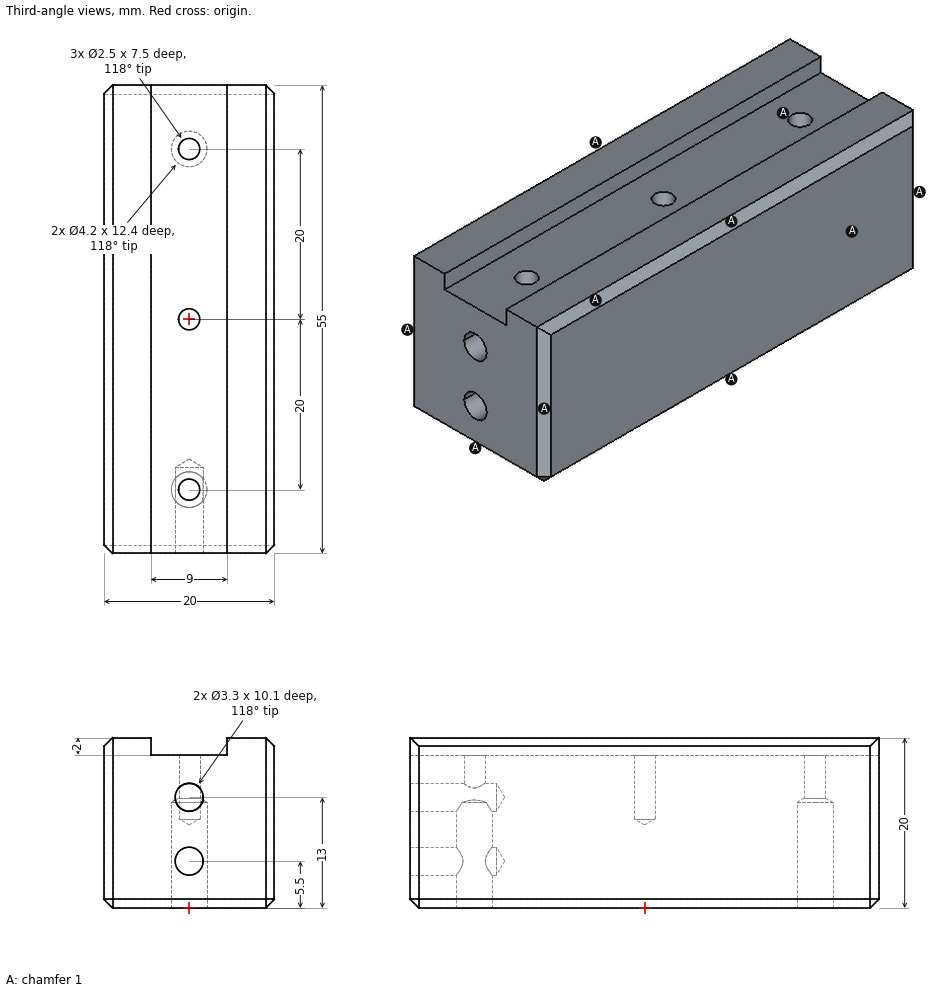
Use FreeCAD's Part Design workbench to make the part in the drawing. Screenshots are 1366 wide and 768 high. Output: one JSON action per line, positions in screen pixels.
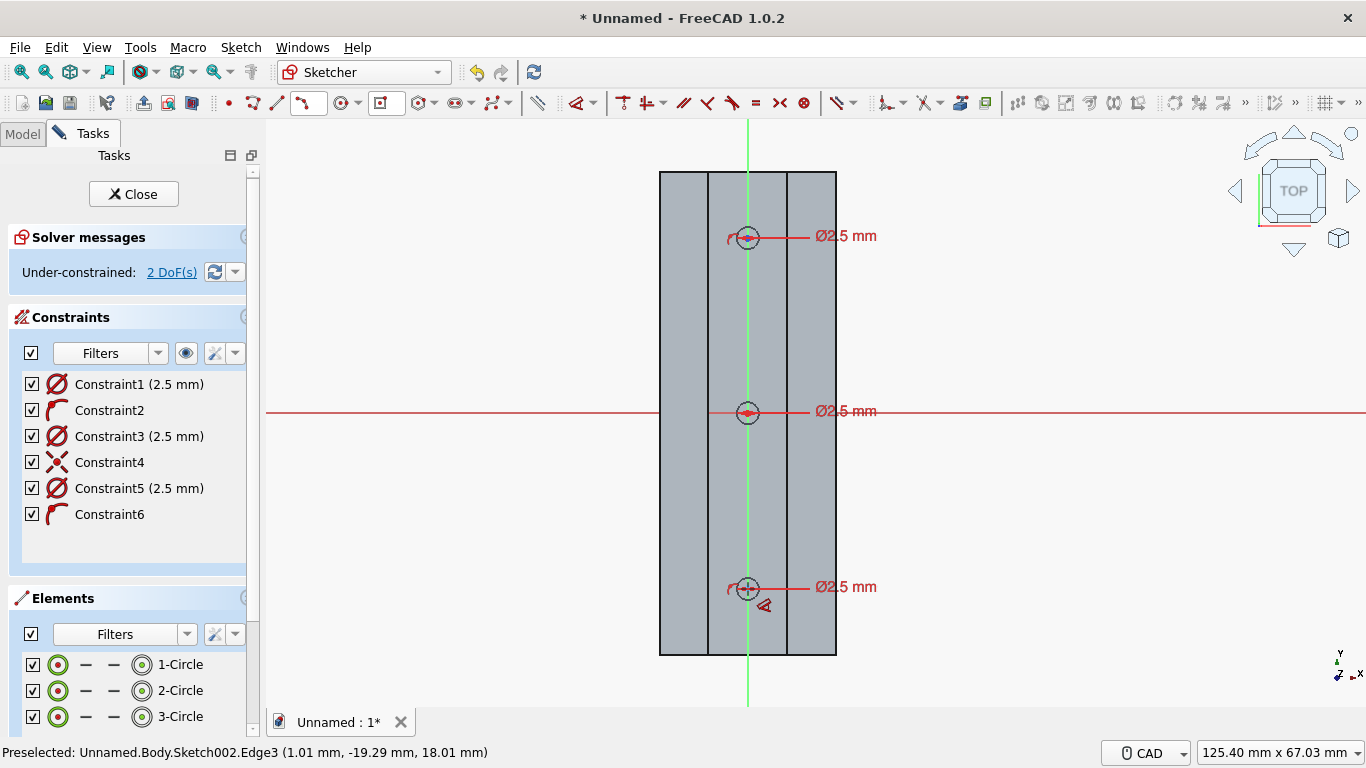
{"action": "left_click", "coordinate": [748, 238]}
{"action": "left_click", "coordinate": [782, 326]}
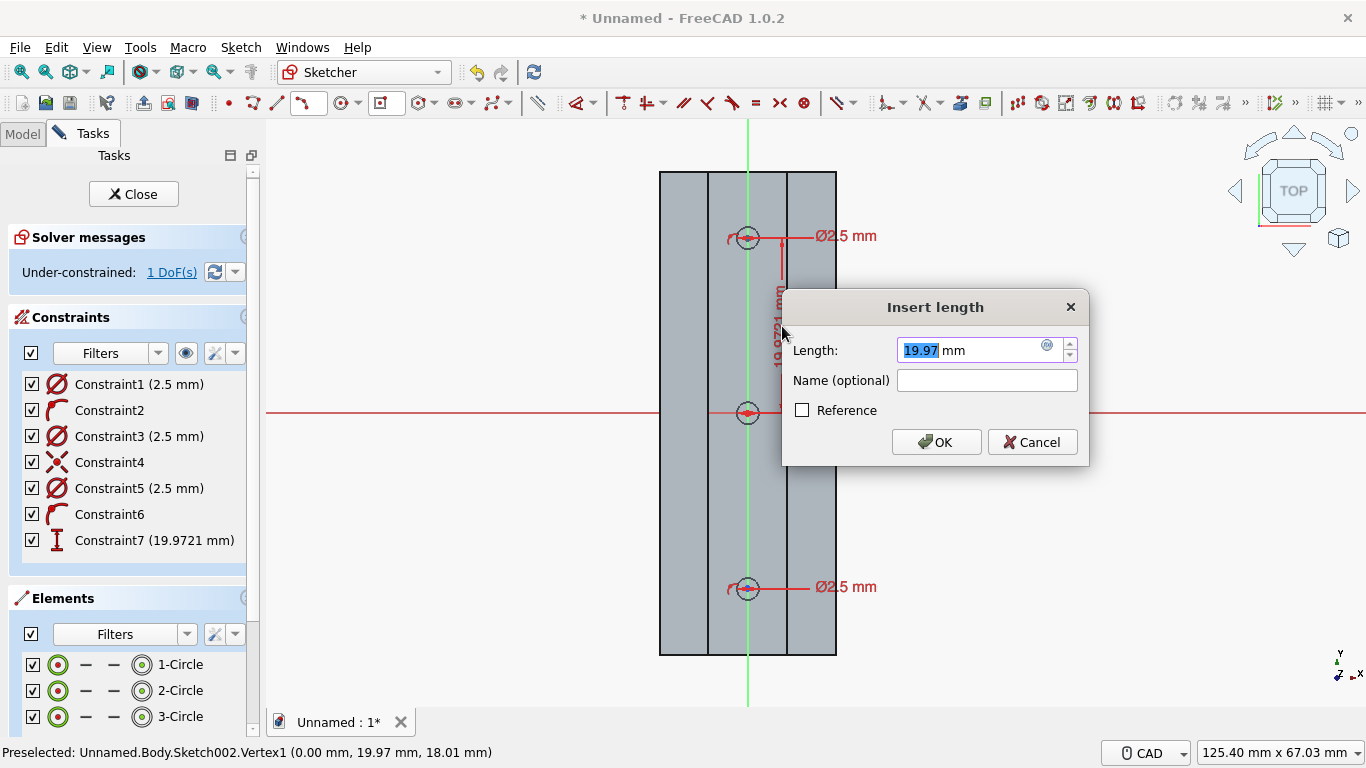
{"action": "type", "text": "20"}
{"action": "key", "text": "Return"}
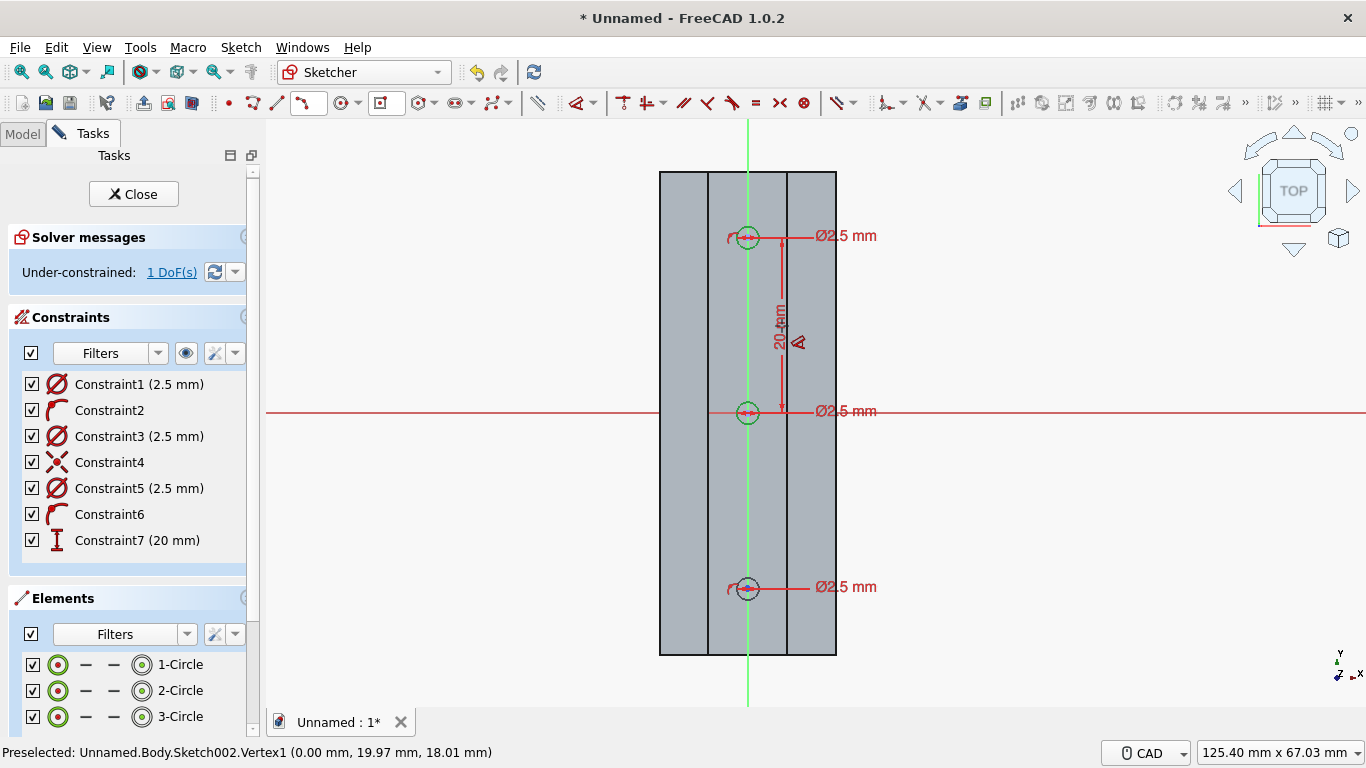
{"action": "left_click", "coordinate": [748, 589]}
{"action": "left_click", "coordinate": [782, 501]}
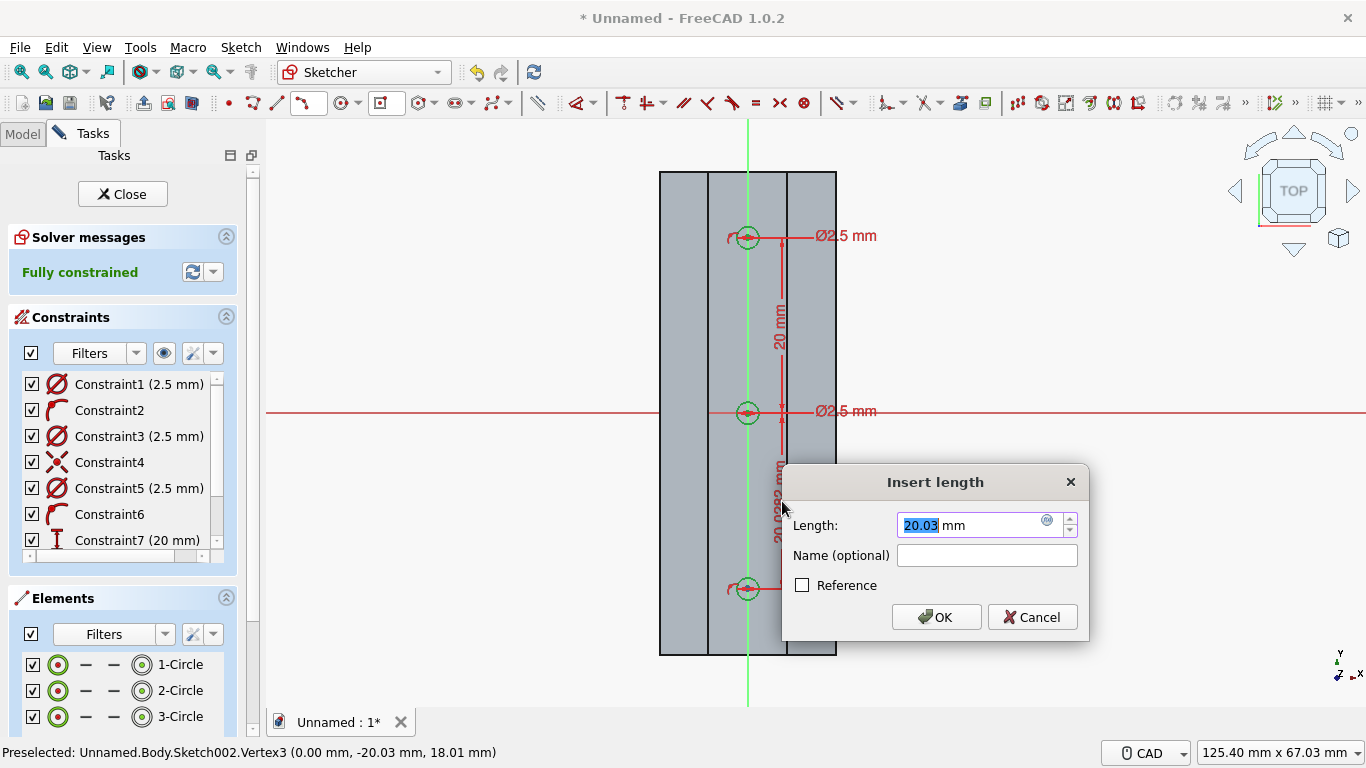
{"action": "type", "text": "20"}
{"action": "key", "text": "Return"}
{"action": "key", "text": "Escape"}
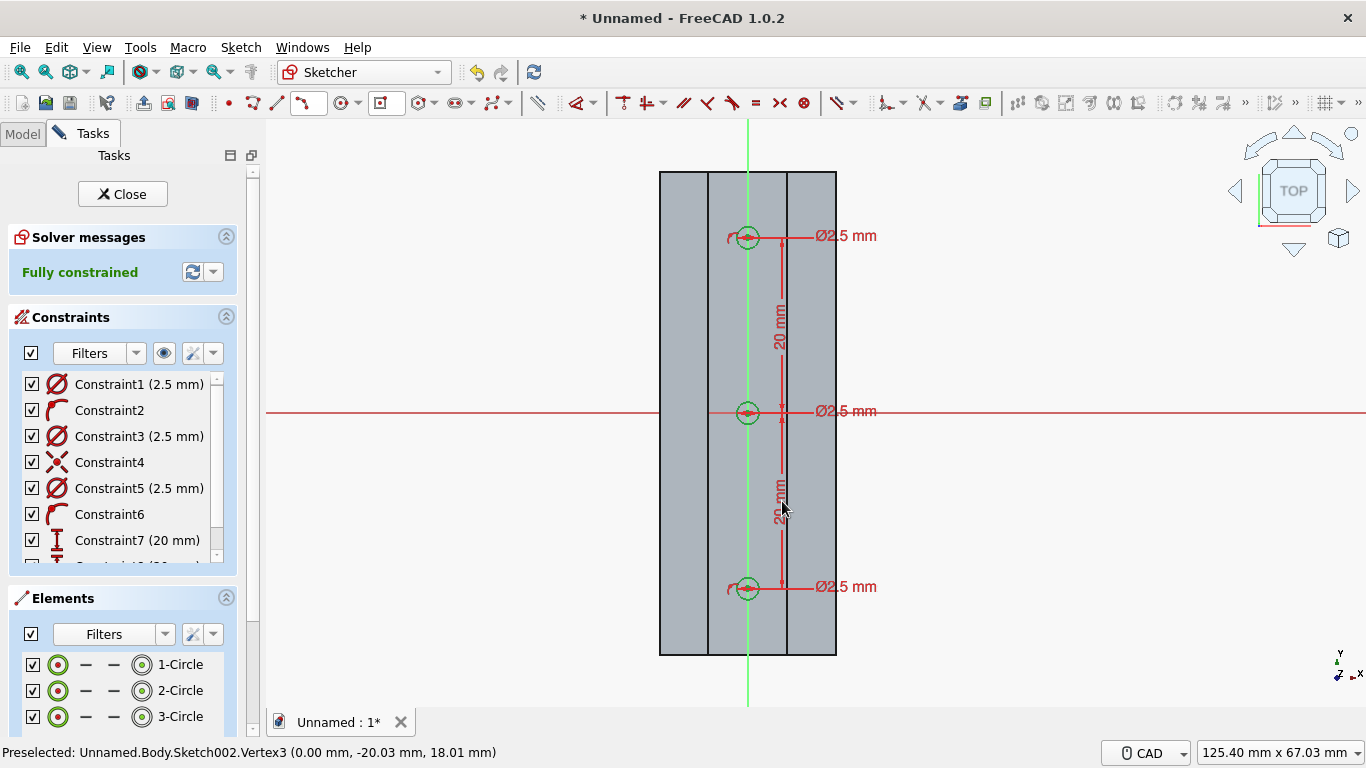
{"action": "left_click", "coordinate": [123, 194]}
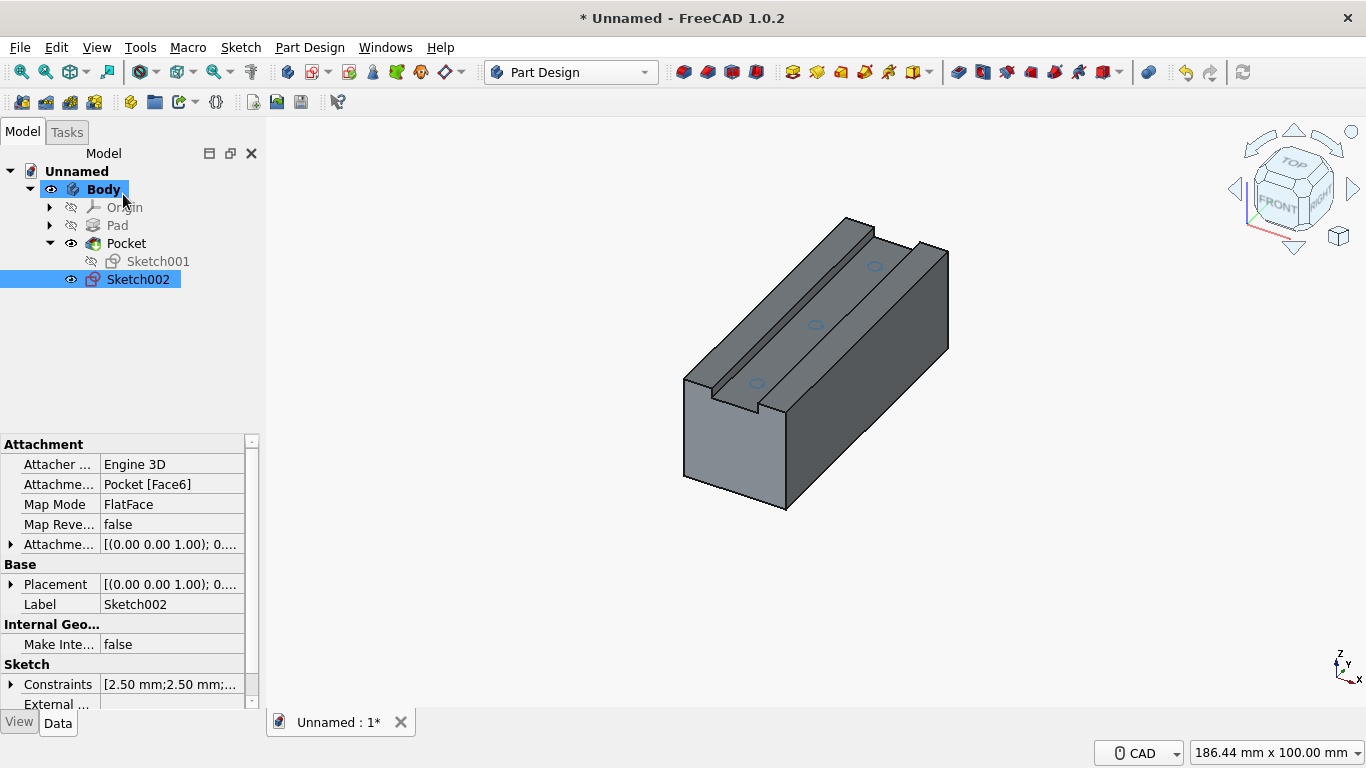
{"action": "left_click", "coordinate": [984, 72]}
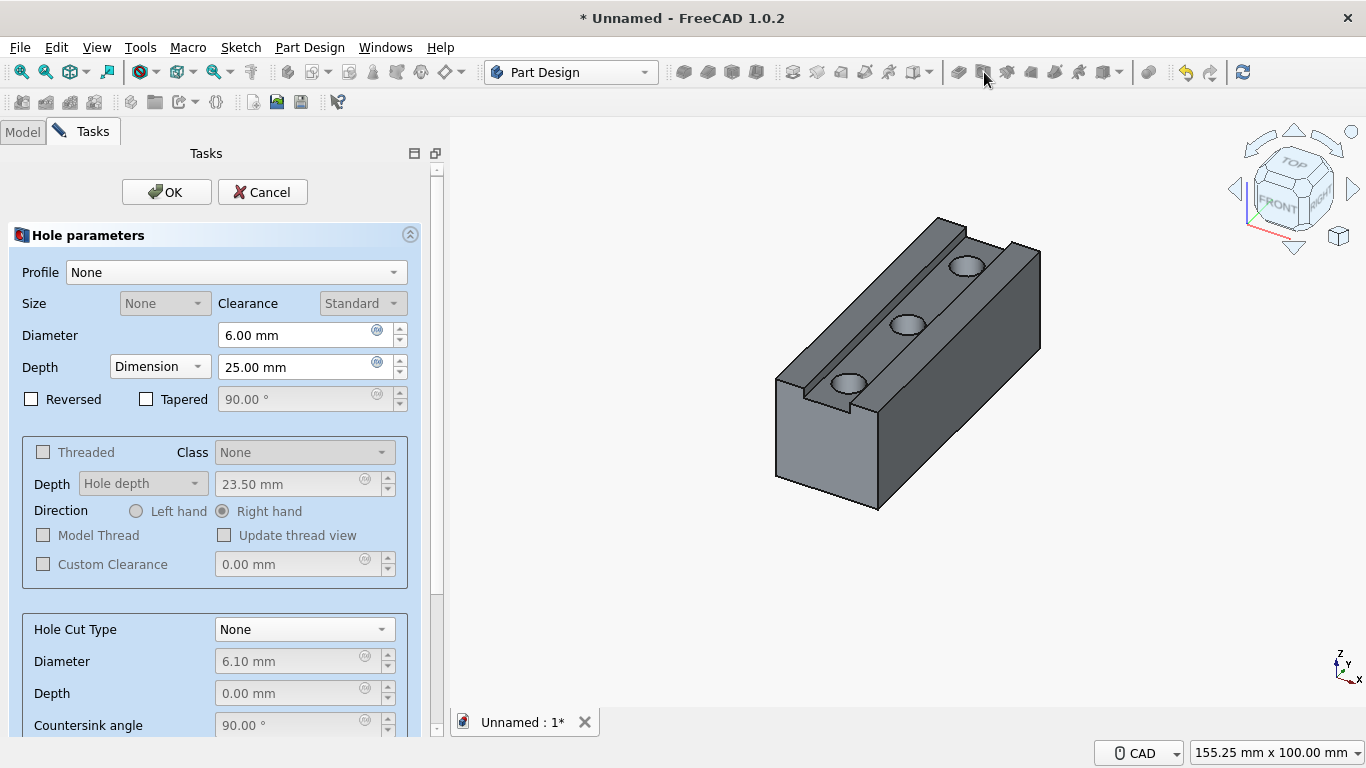
{"action": "triple_click", "coordinate": [305, 335]}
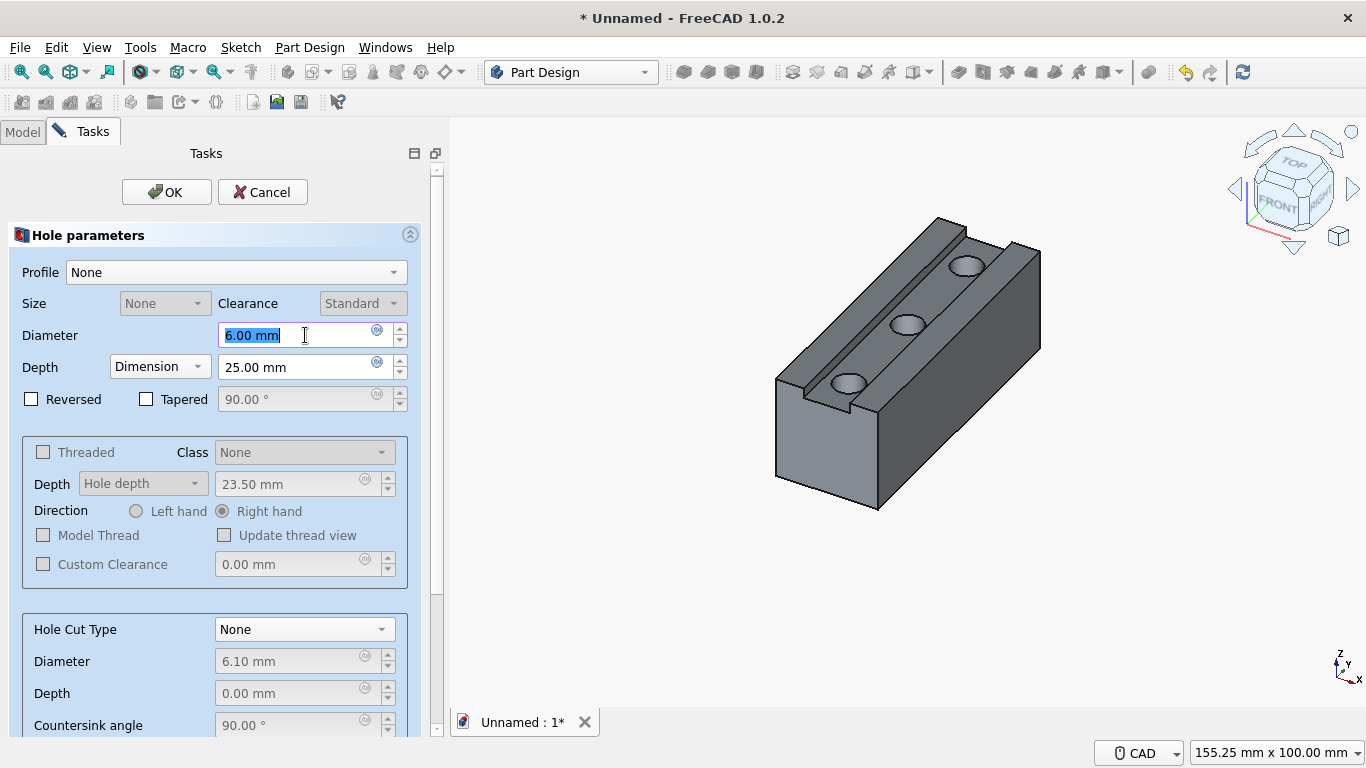
{"action": "type", "text": "2.5"}
{"action": "key", "text": "Tab"}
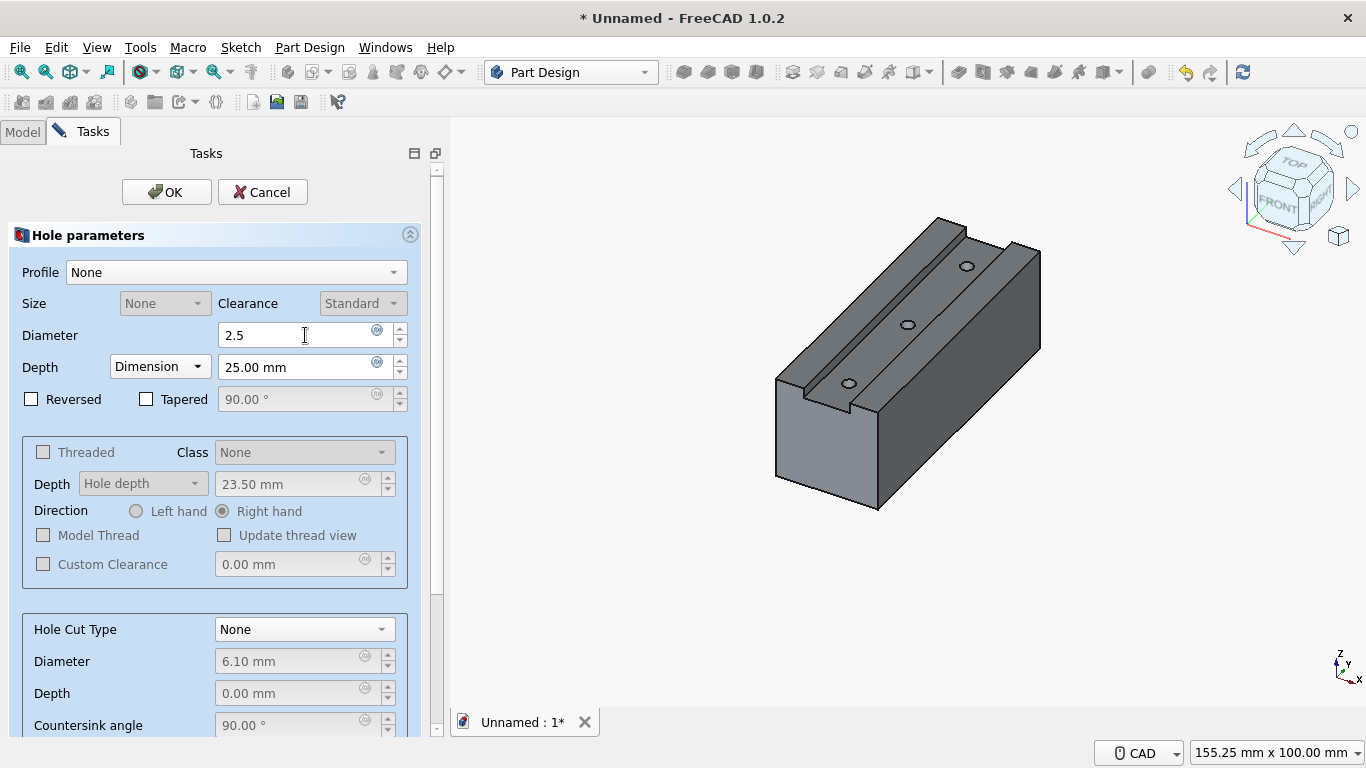
{"action": "triple_click", "coordinate": [305, 367]}